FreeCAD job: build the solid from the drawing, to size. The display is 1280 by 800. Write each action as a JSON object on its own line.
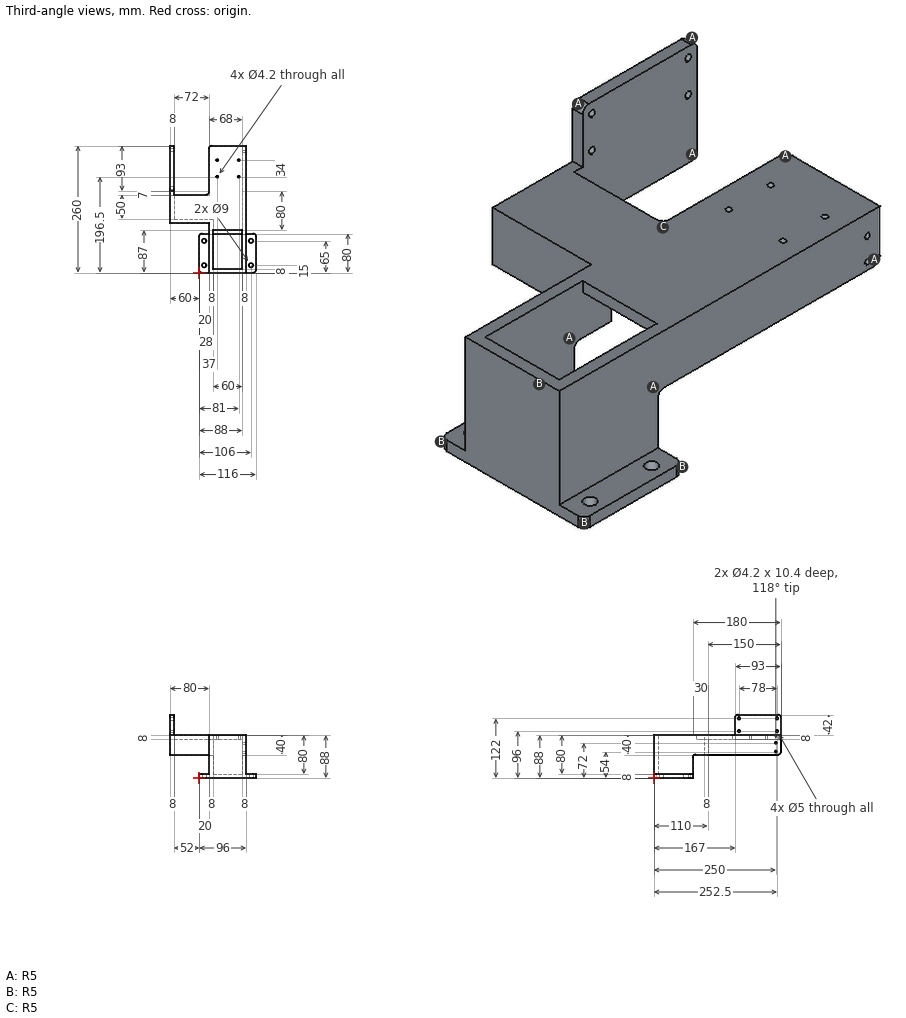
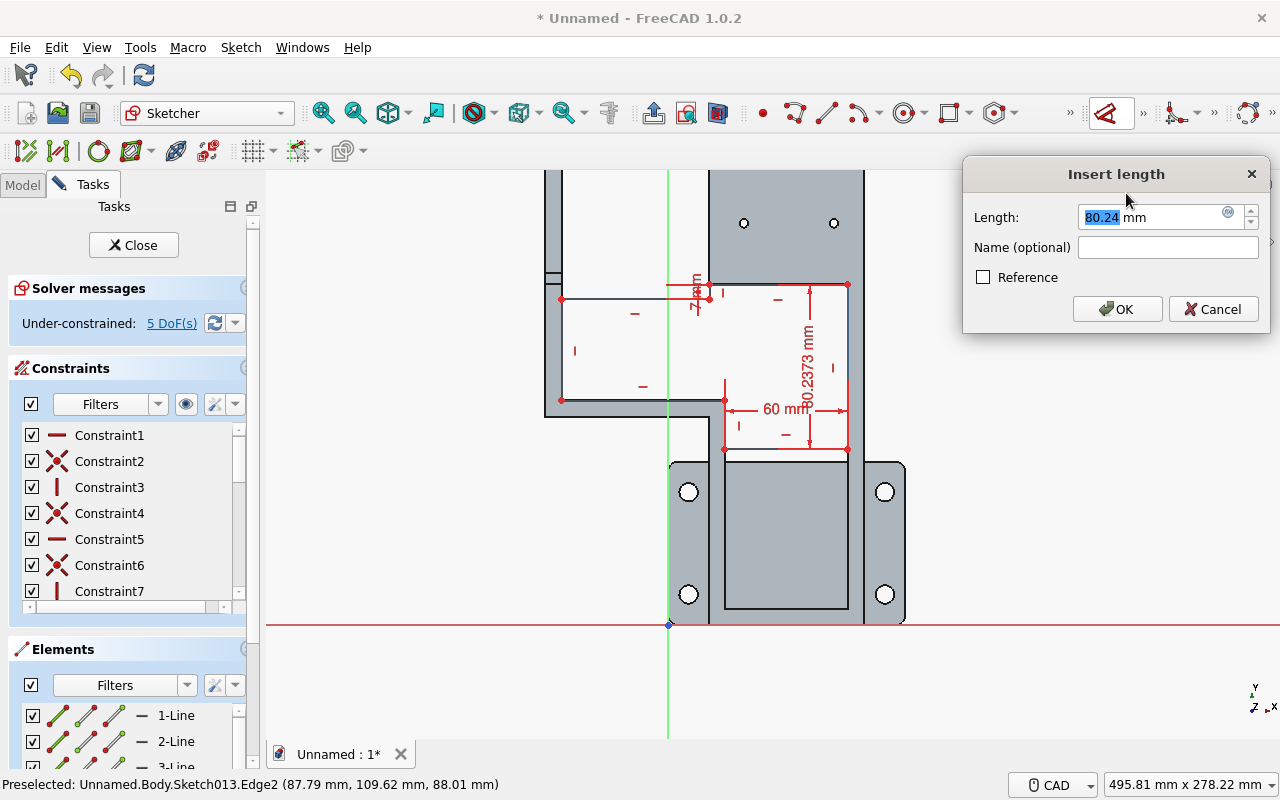
{"action": "type", "text": "80"}
{"action": "key", "text": "Return"}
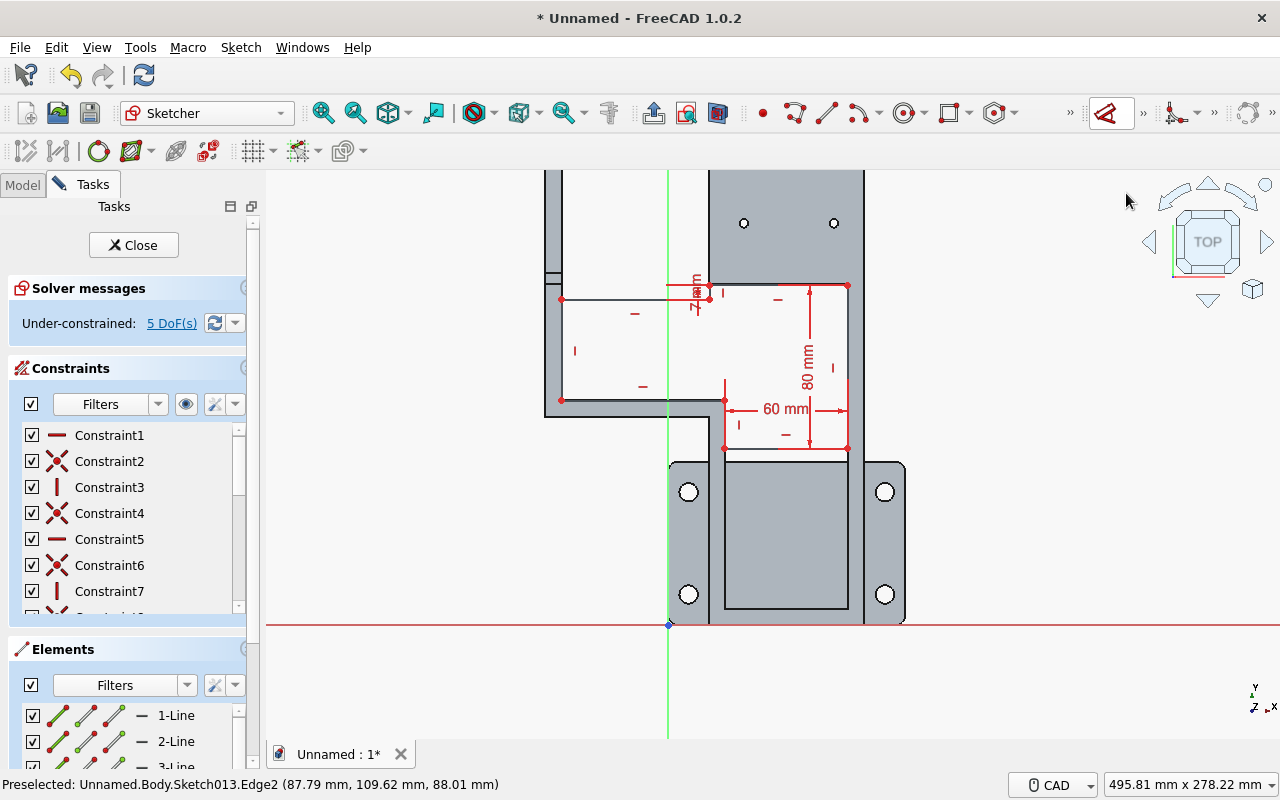
{"action": "left_click", "coordinate": [806, 285]}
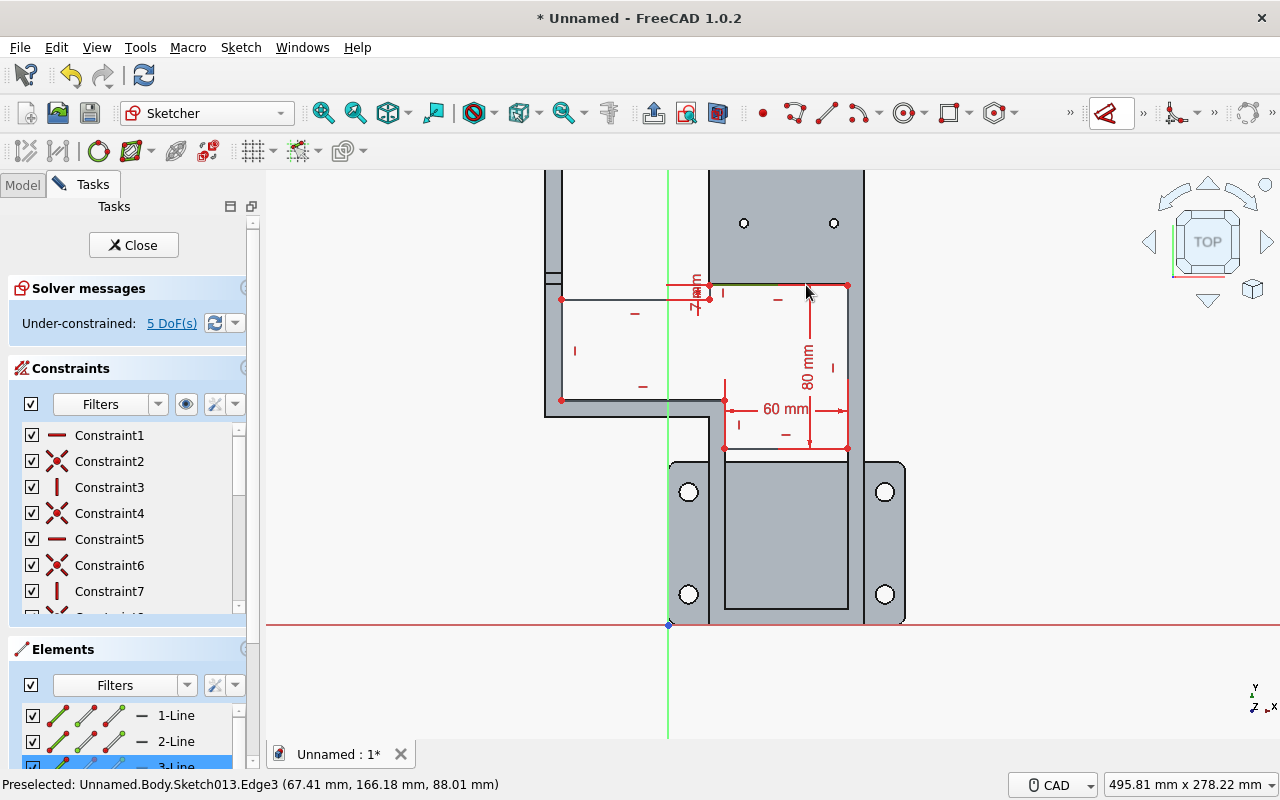
{"action": "left_click", "coordinate": [1128, 114]}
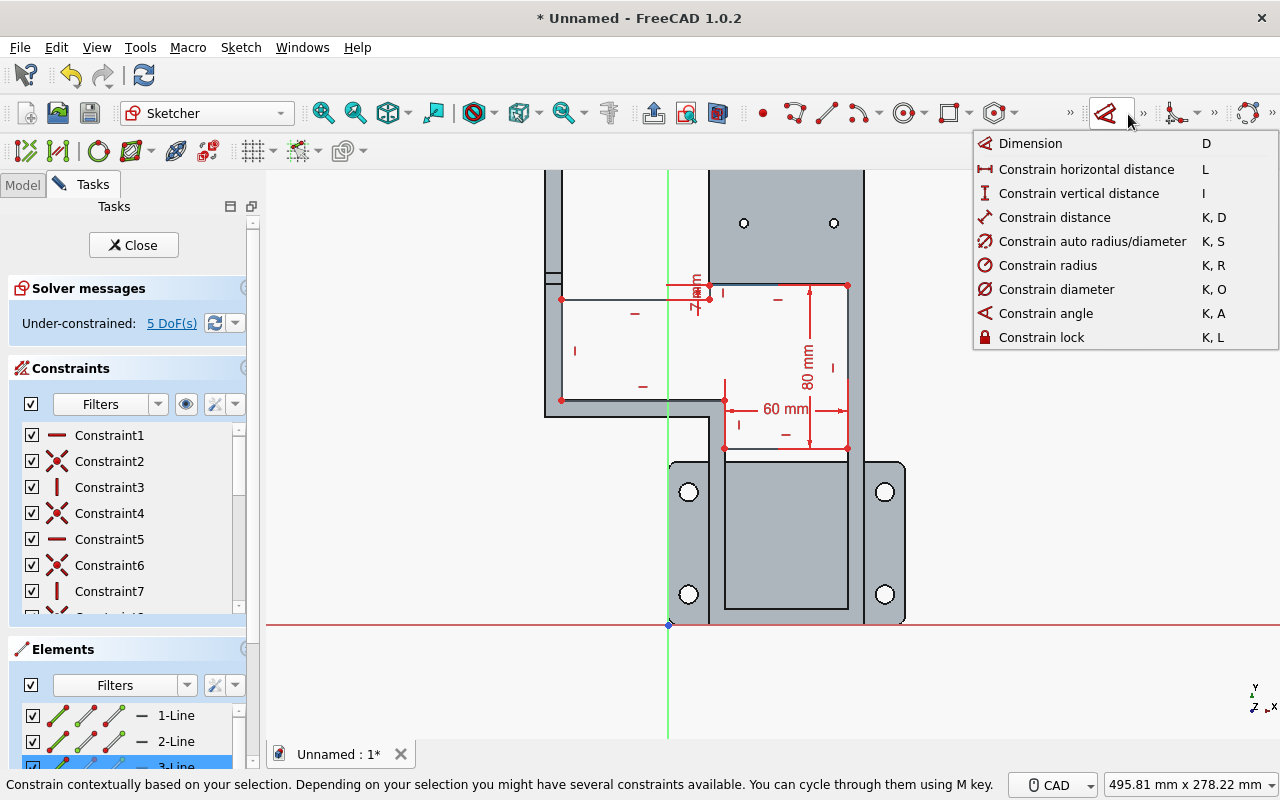
{"action": "left_click", "coordinate": [1126, 169]}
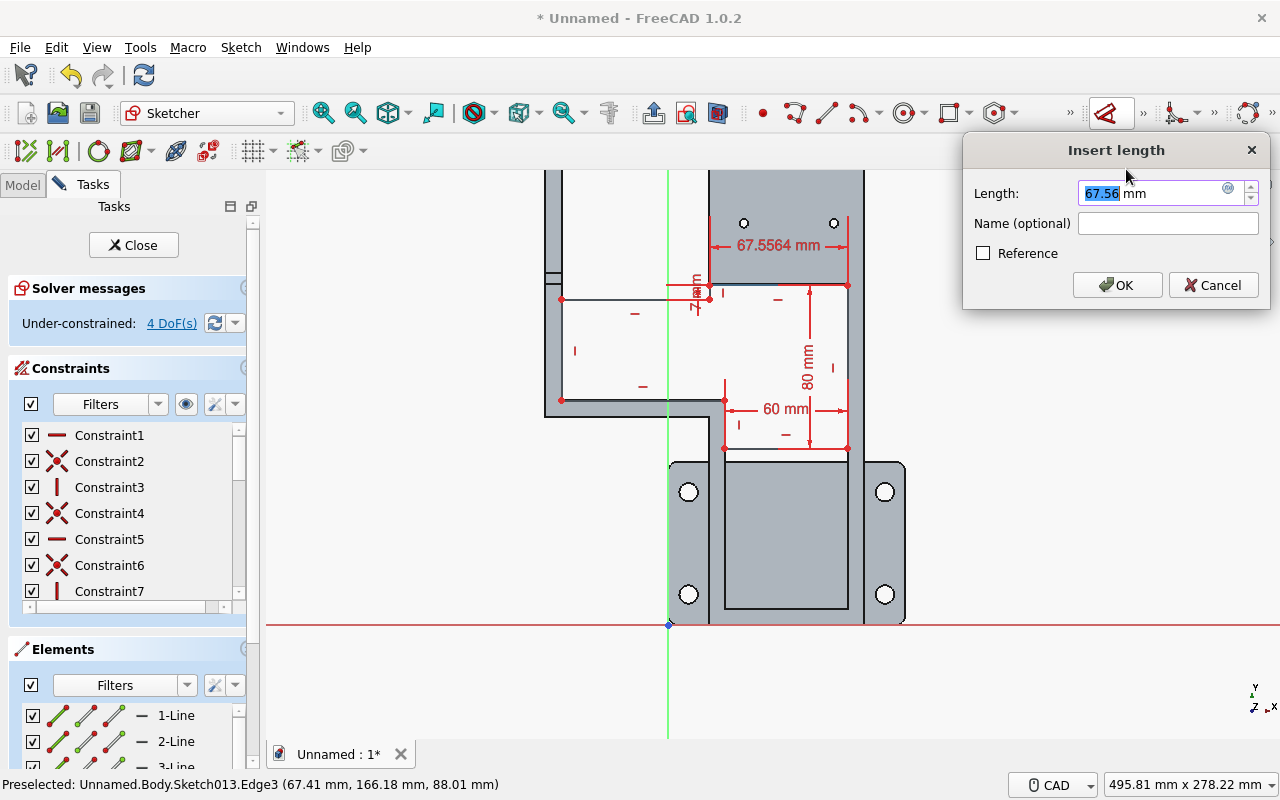
{"action": "type", "text": "68"}
{"action": "key", "text": "Return"}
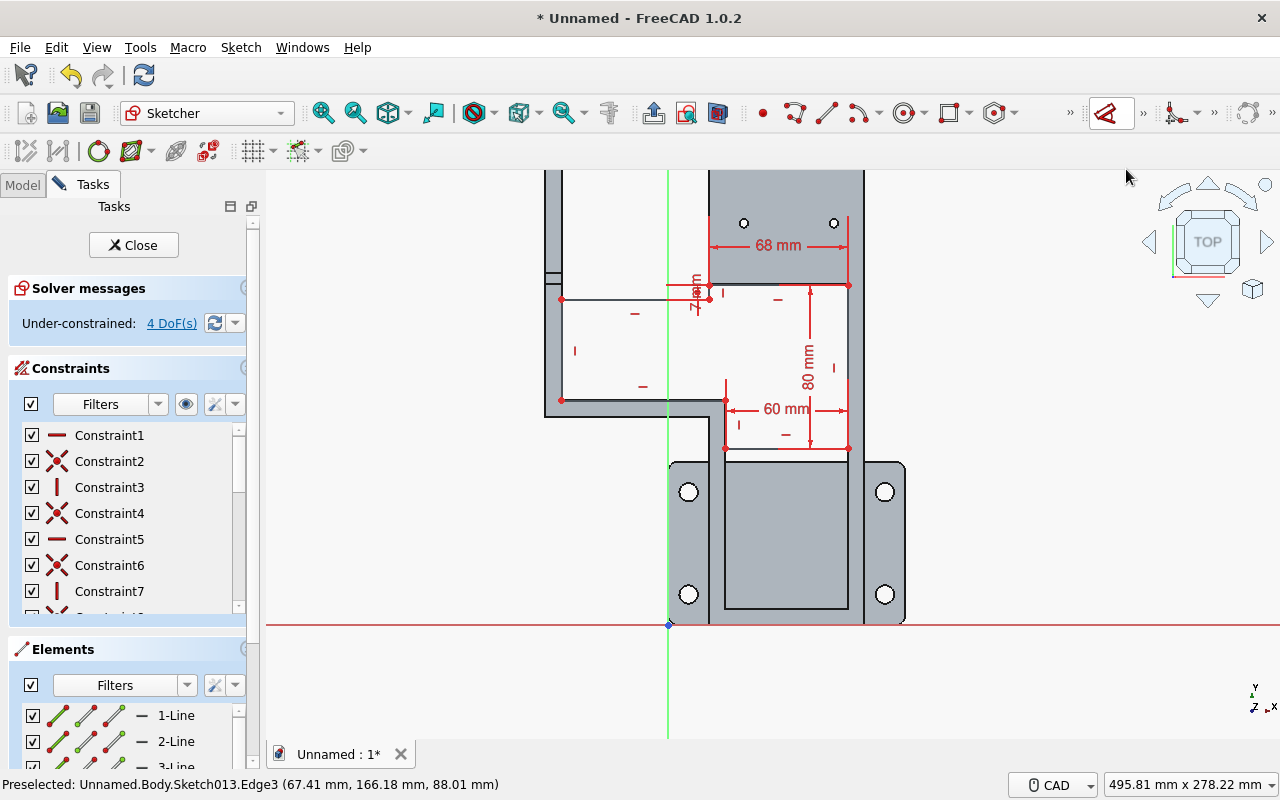
{"action": "left_click", "coordinate": [665, 300]}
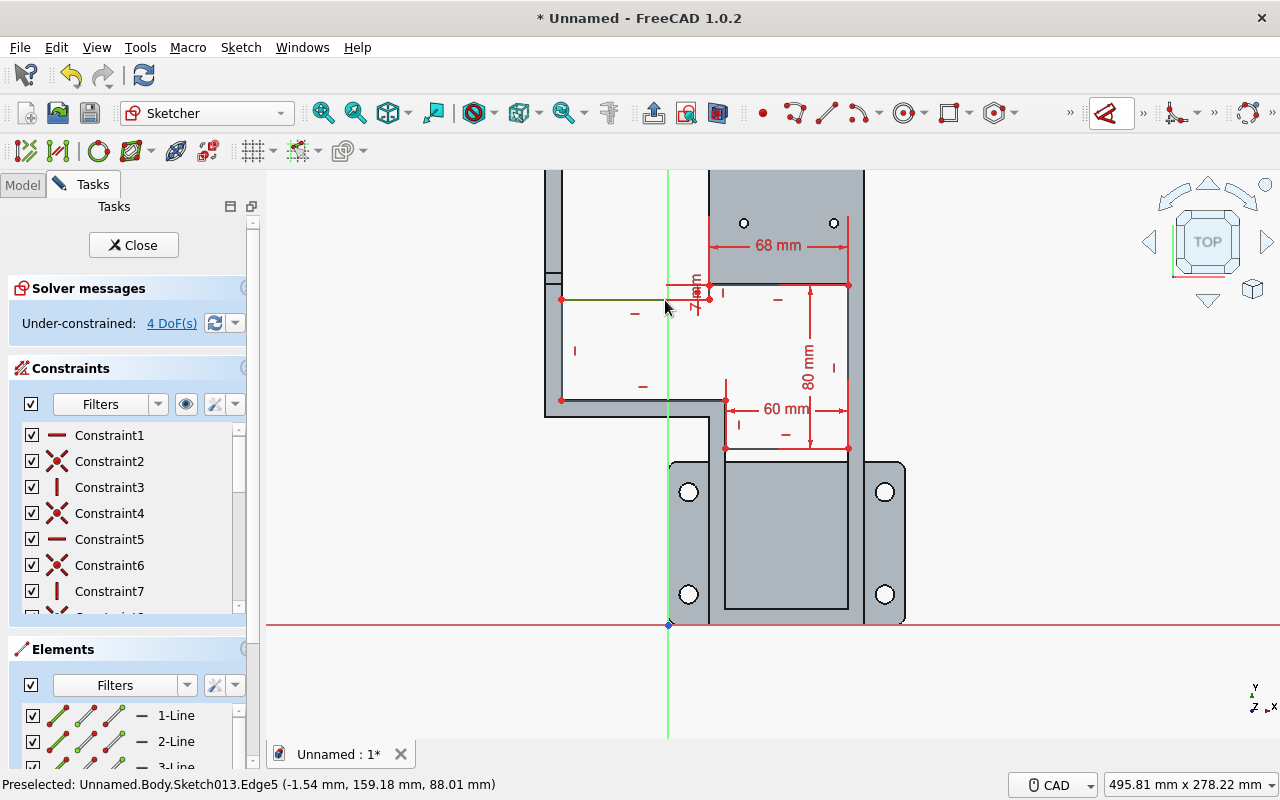
{"action": "left_click", "coordinate": [1128, 114]}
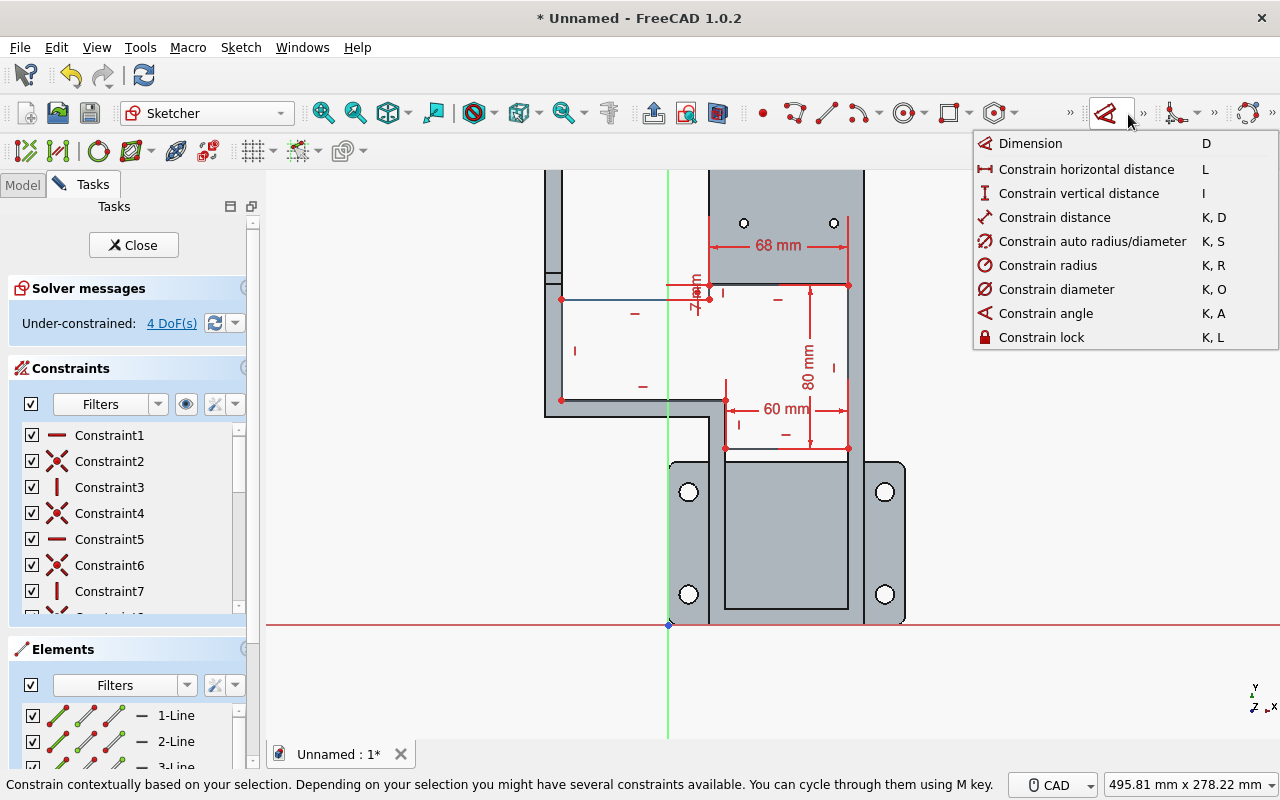
{"action": "left_click", "coordinate": [1126, 169]}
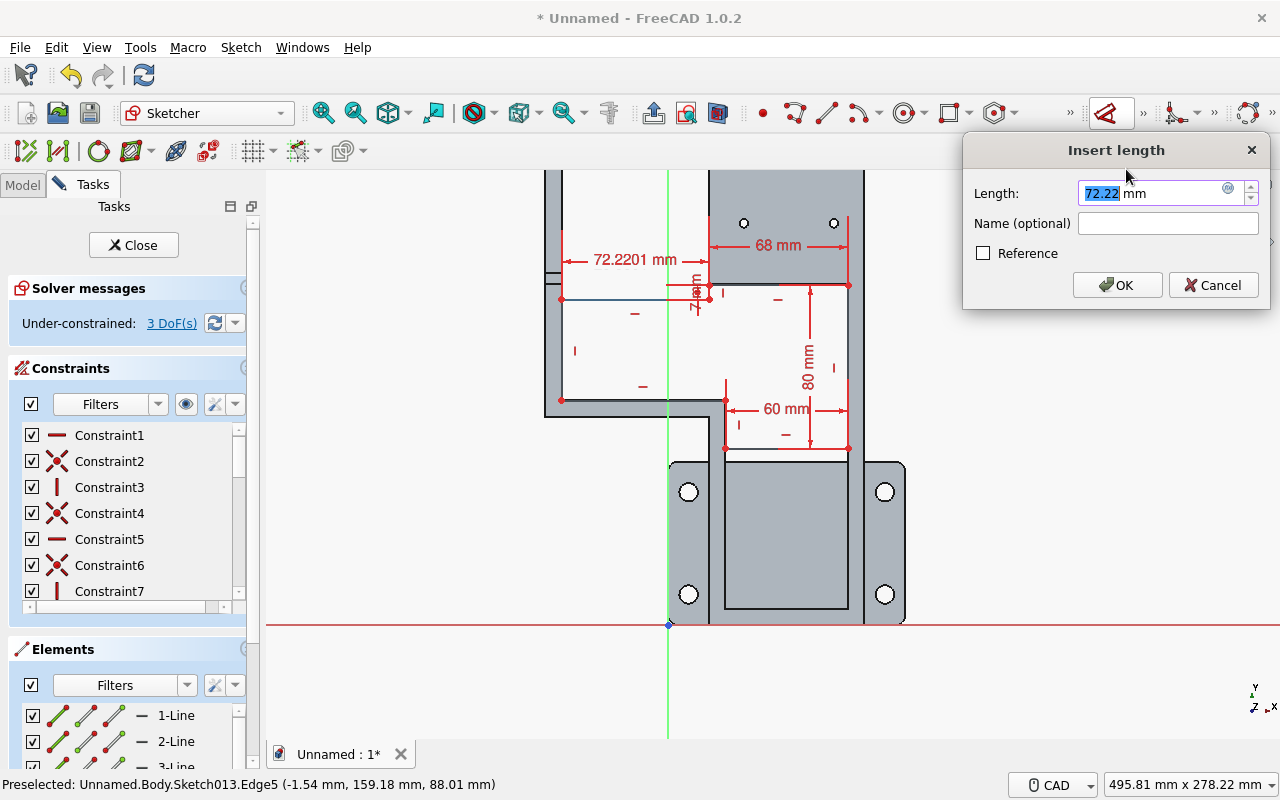
{"action": "type", "text": "72"}
{"action": "key", "text": "Return"}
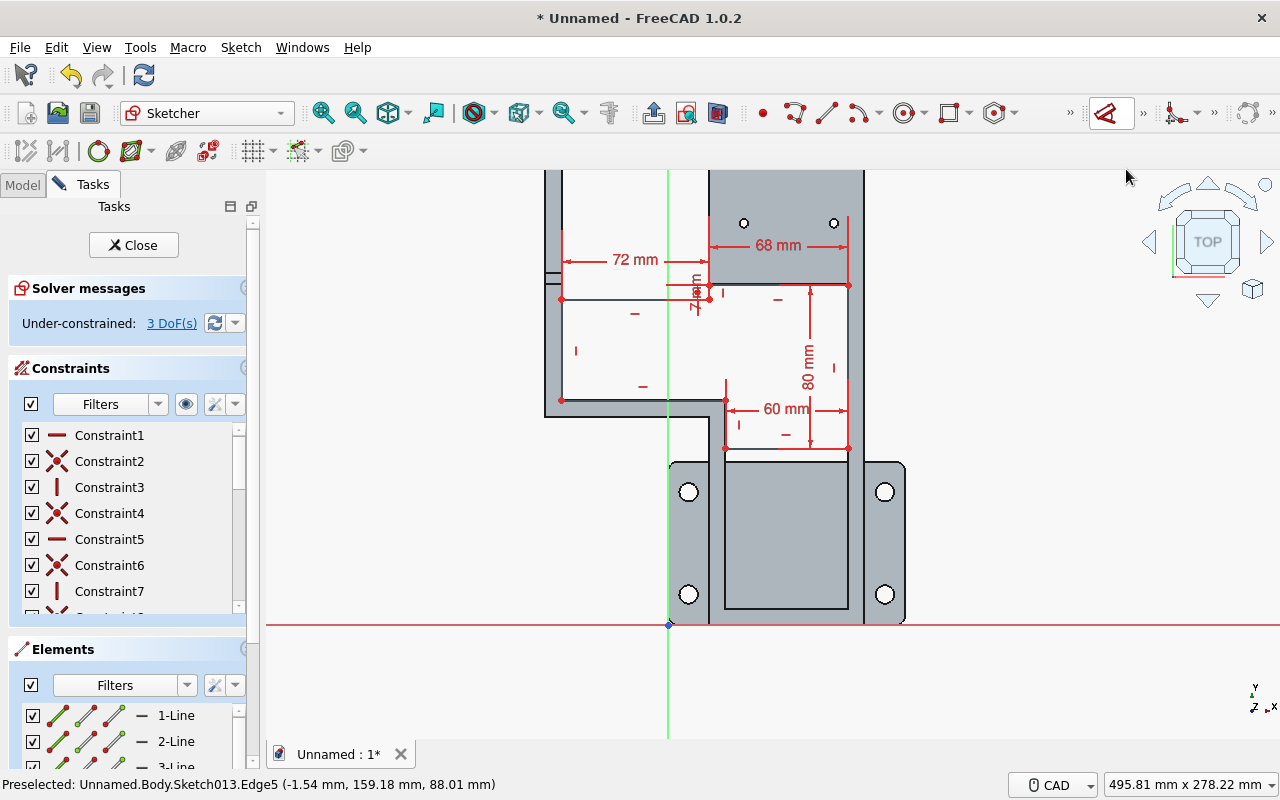
{"action": "left_click", "coordinate": [562, 330]}